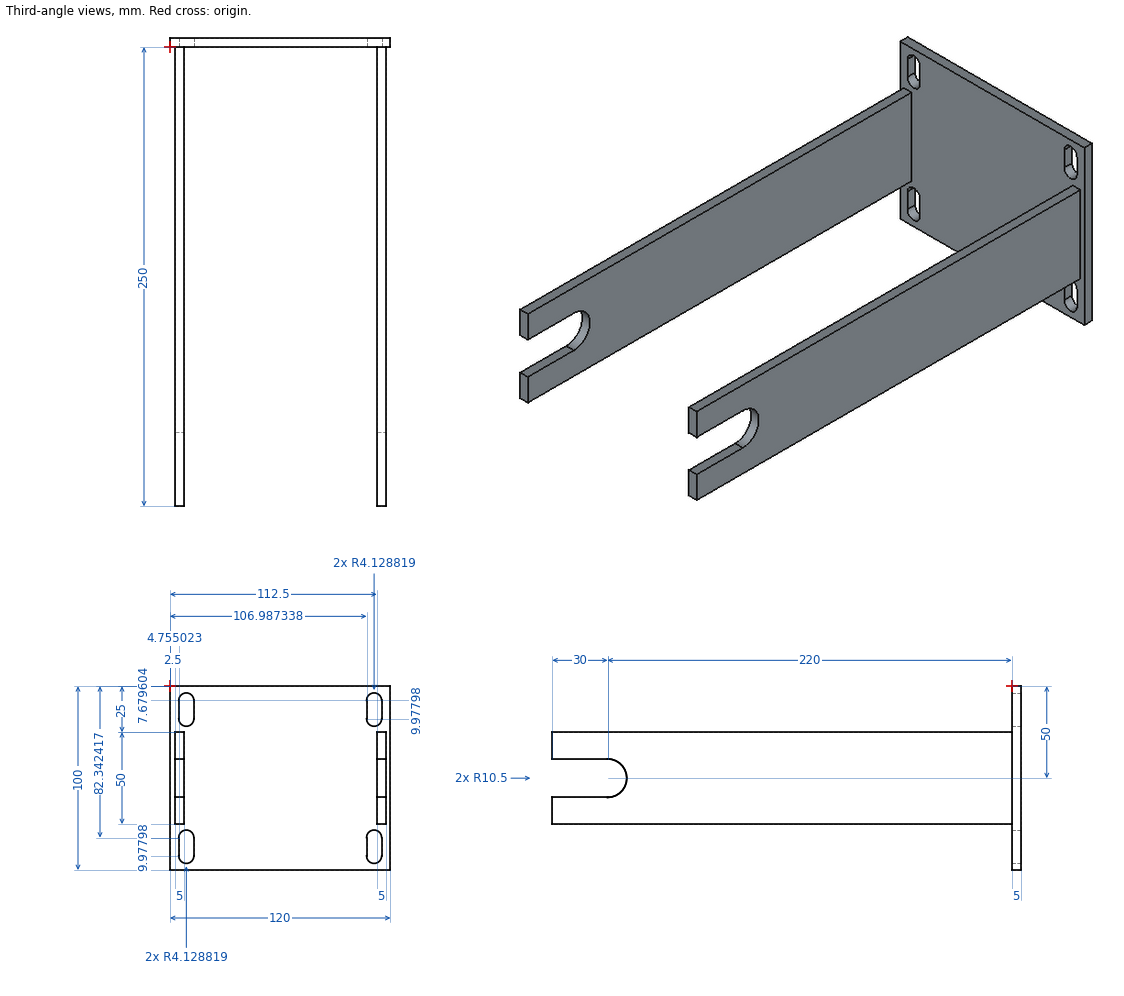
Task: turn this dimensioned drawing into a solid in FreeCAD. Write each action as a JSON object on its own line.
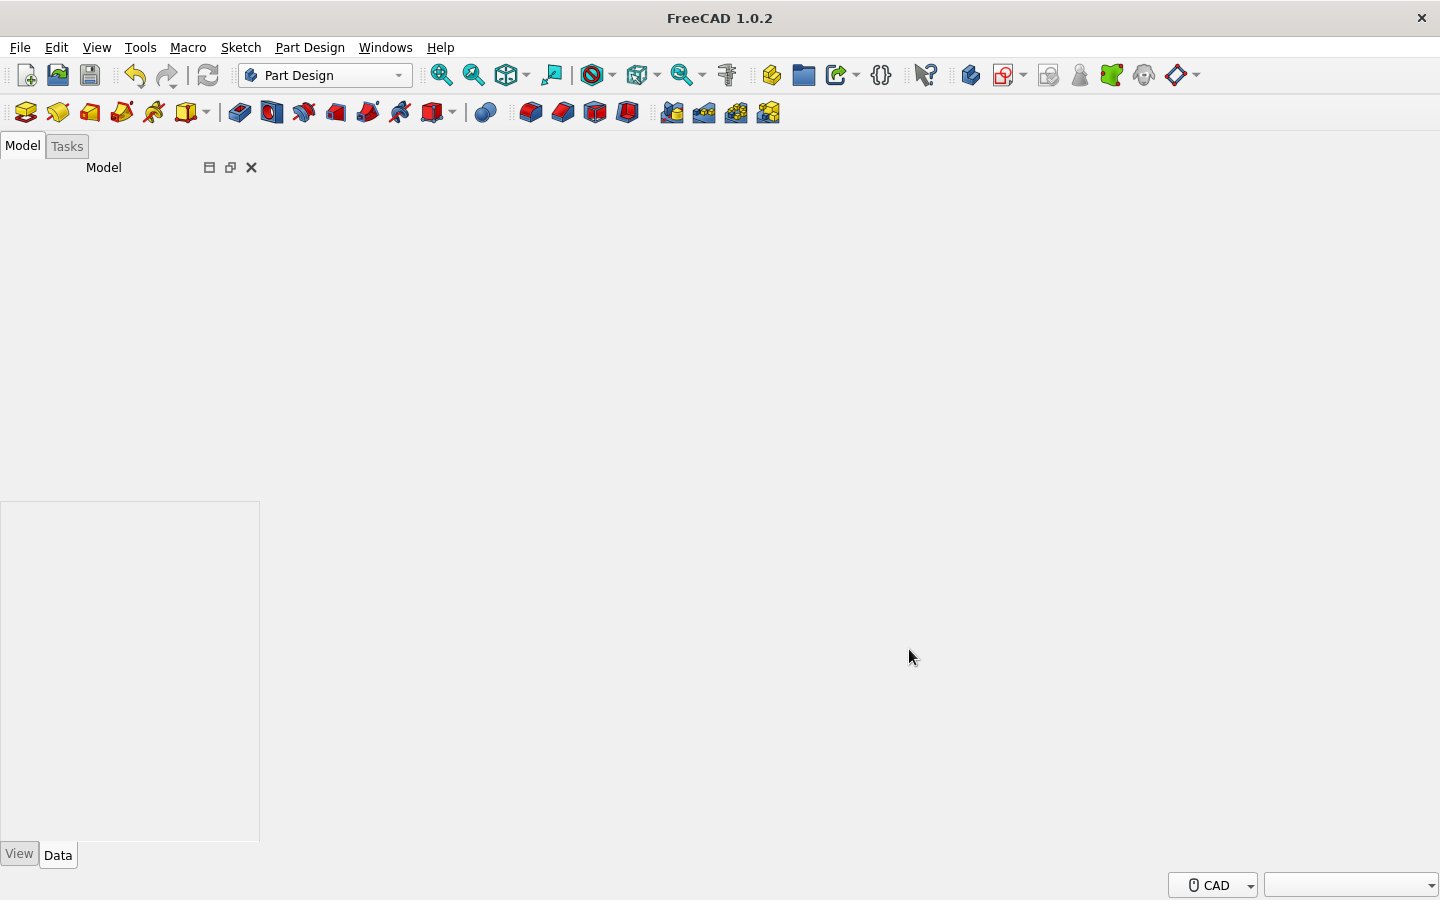
{"action": "left_click", "coordinate": [26, 76]}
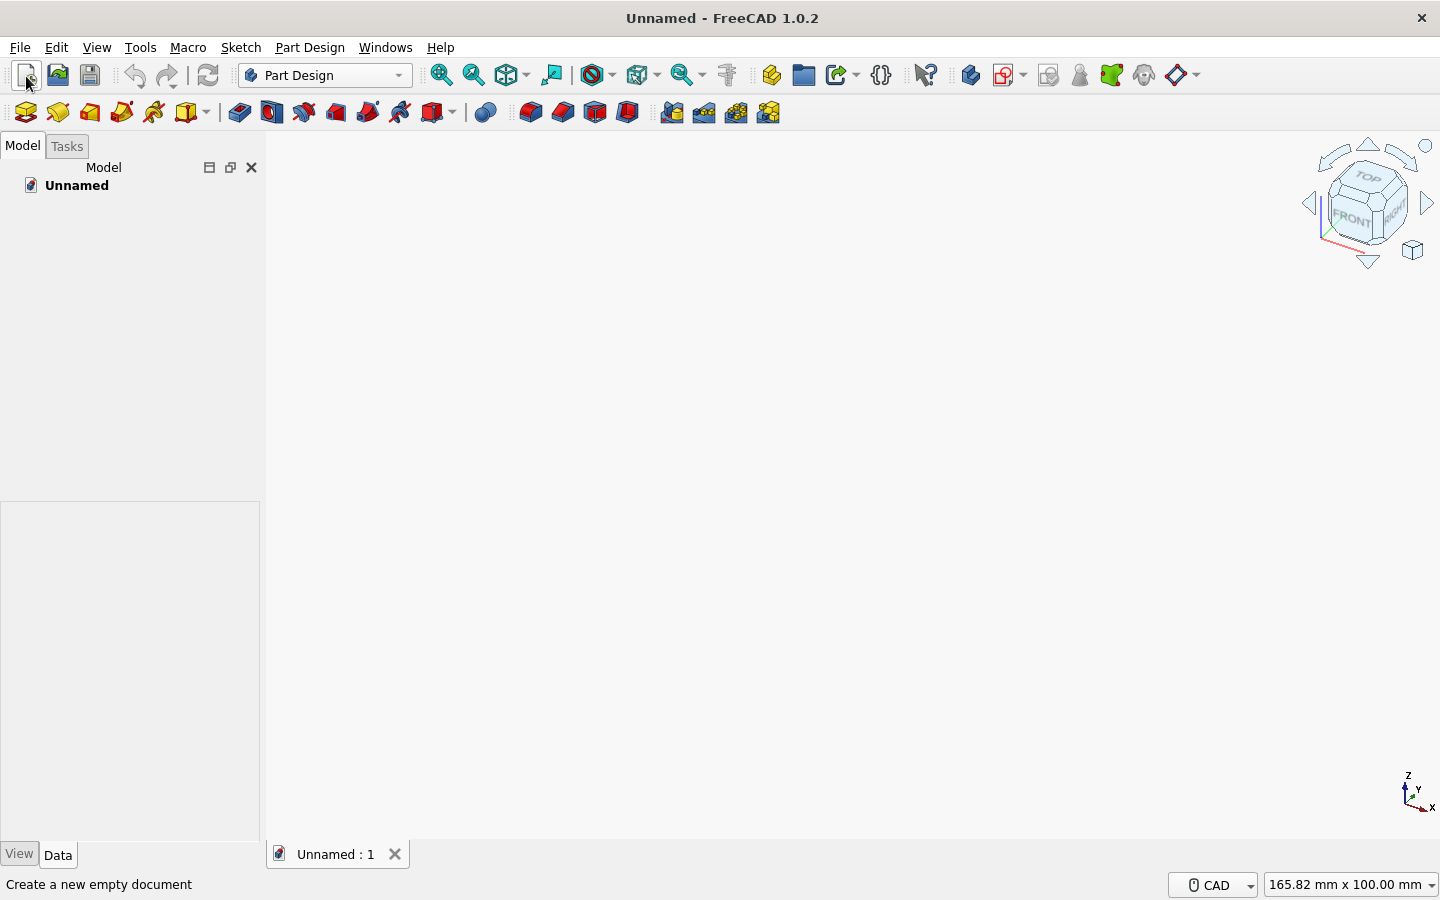
{"action": "left_click", "coordinate": [1004, 76]}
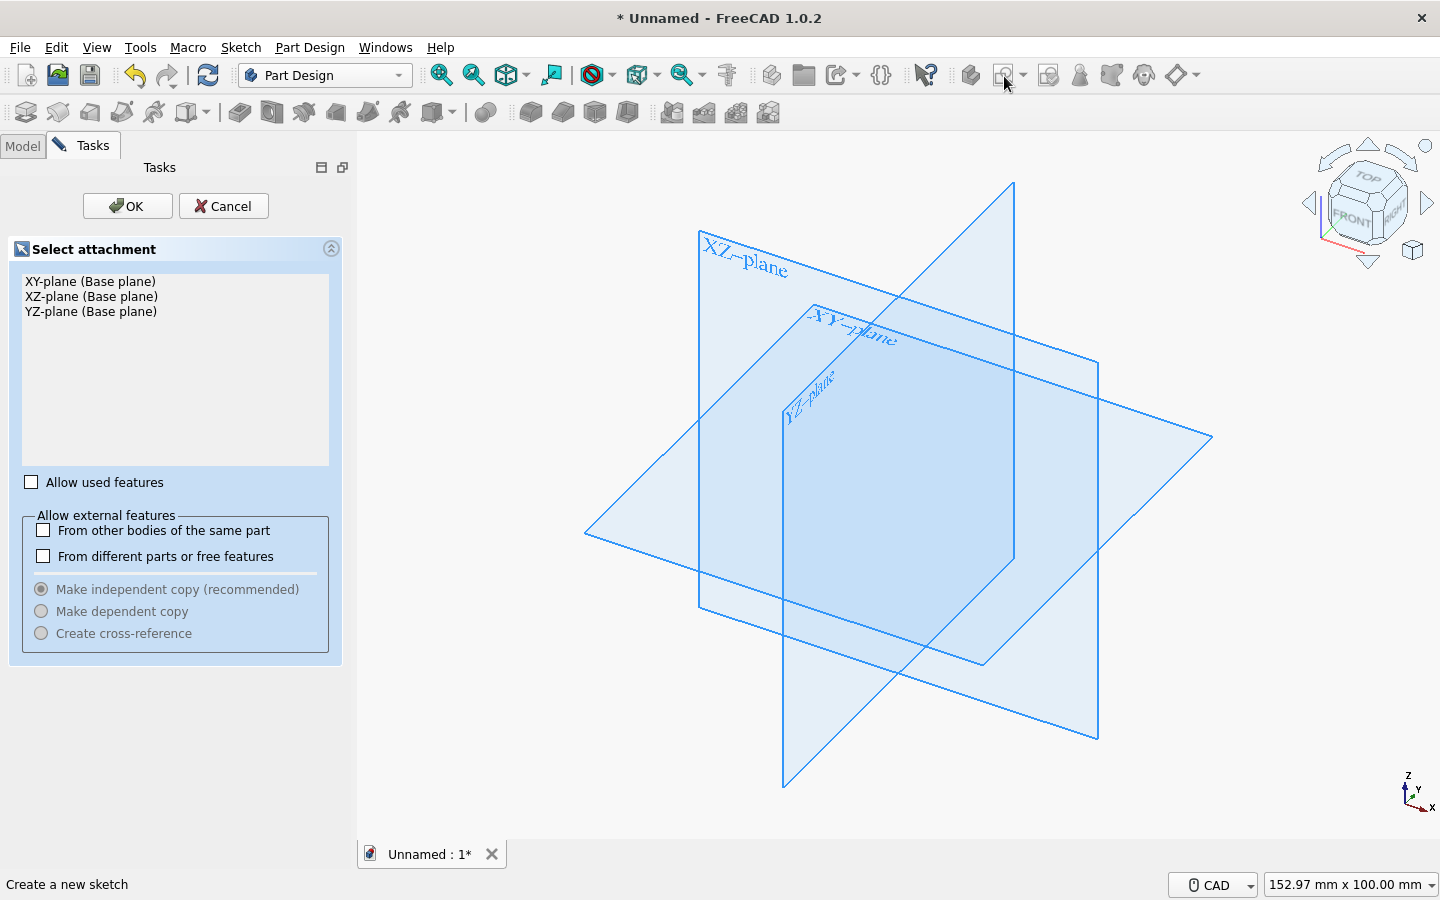
{"action": "left_click", "coordinate": [82, 296]}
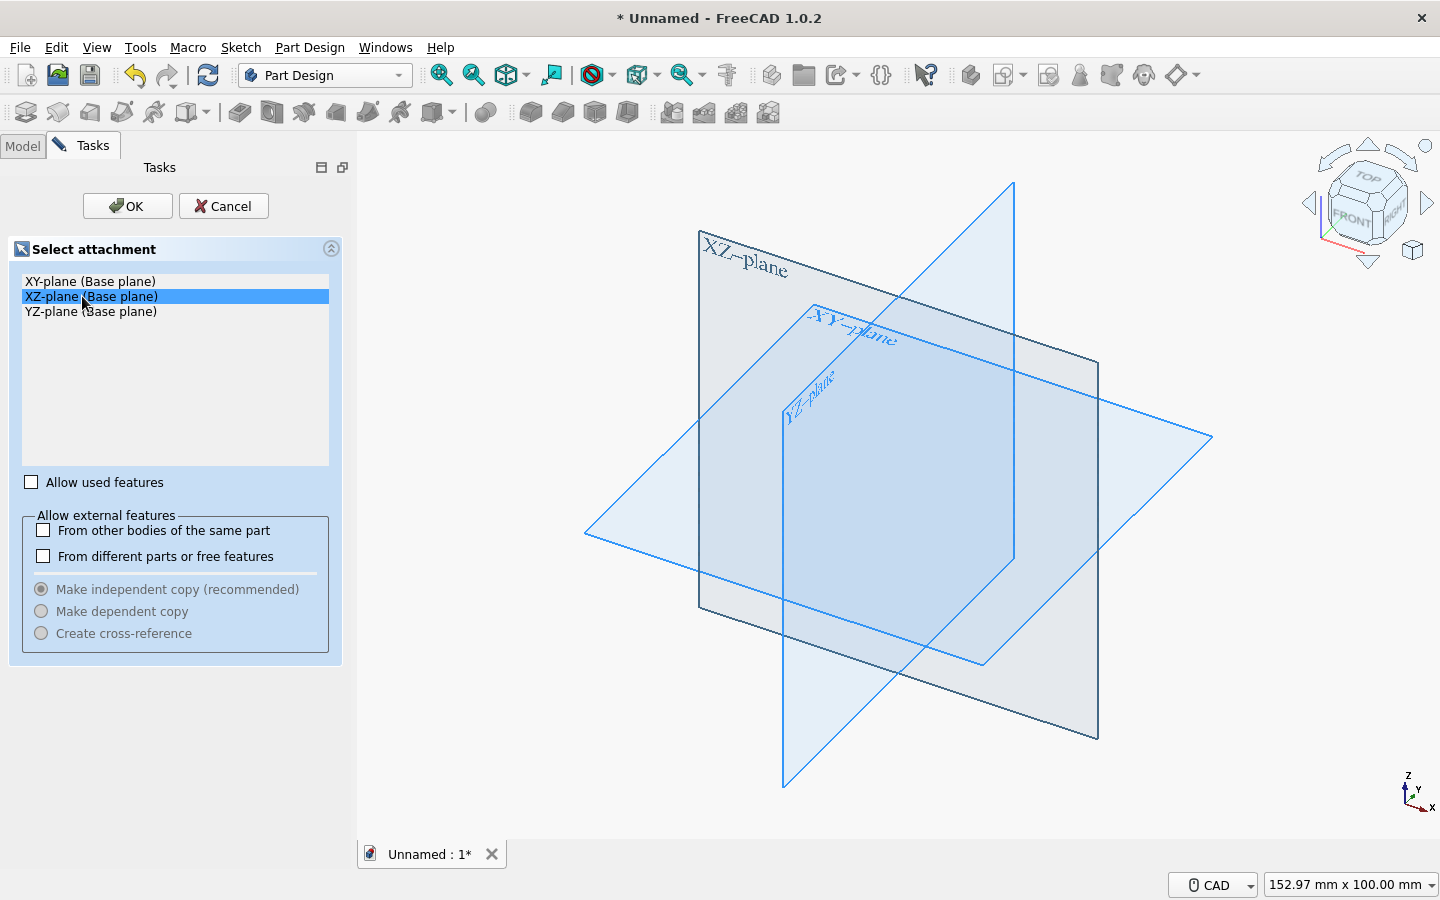
{"action": "left_click", "coordinate": [128, 206]}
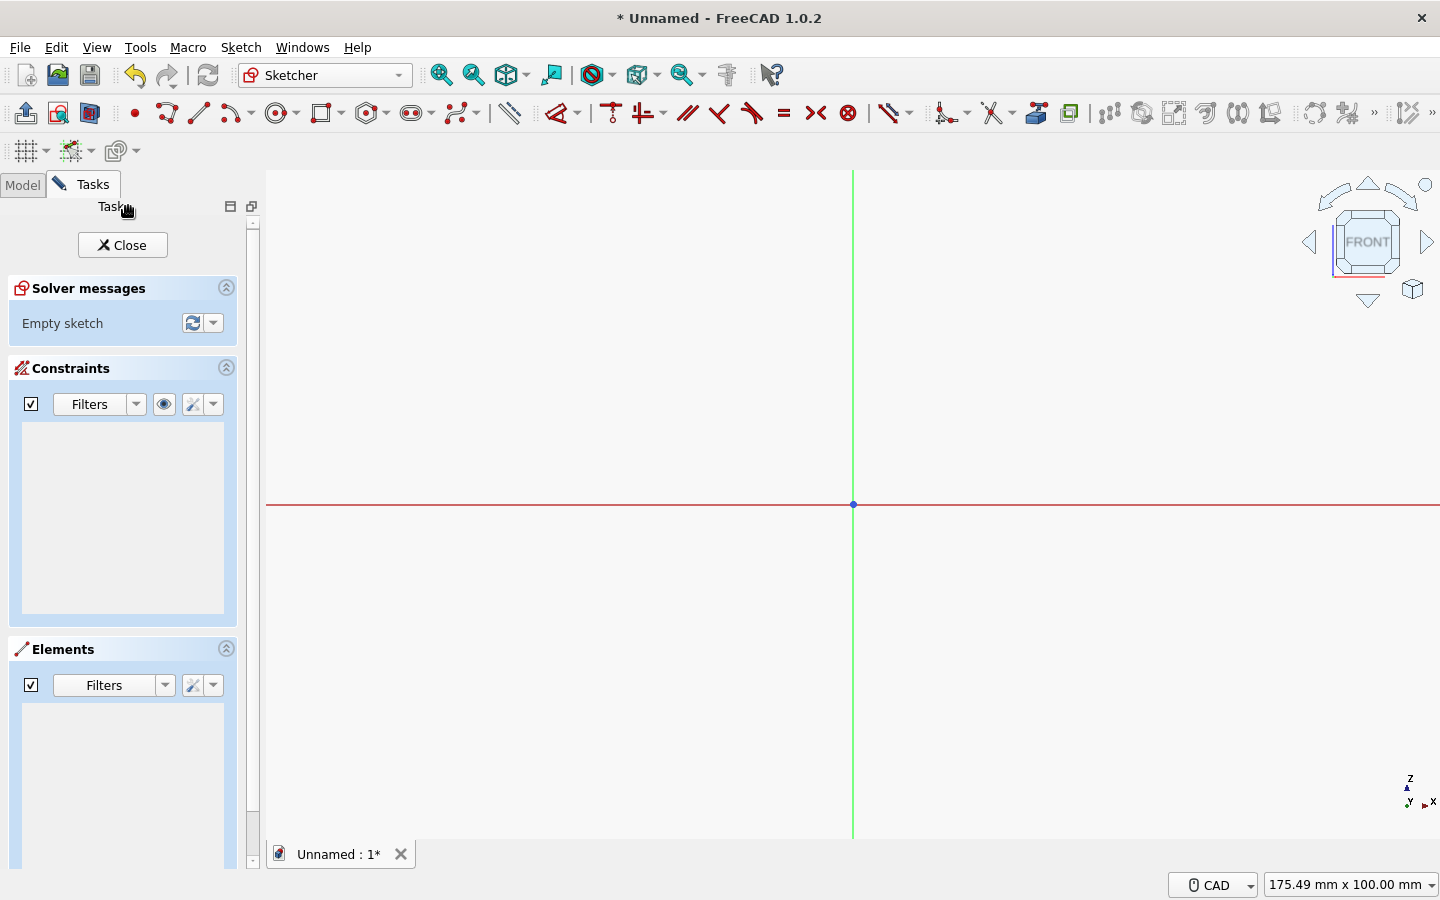
{"action": "scroll", "coordinate": [294, 198], "scroll_direction": "down", "scroll_amount": 3}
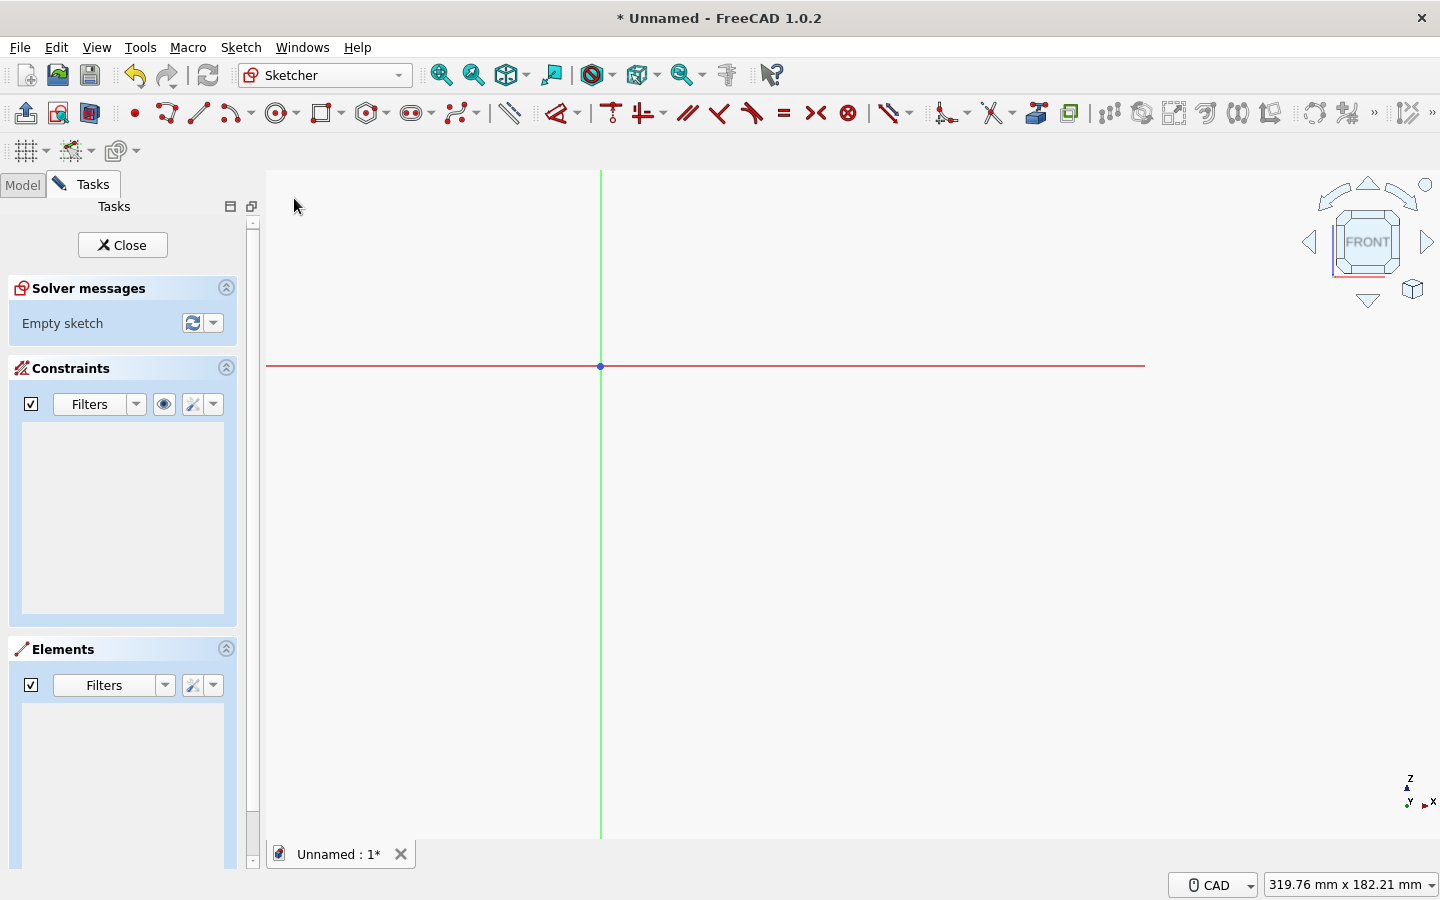
{"action": "left_click", "coordinate": [322, 114]}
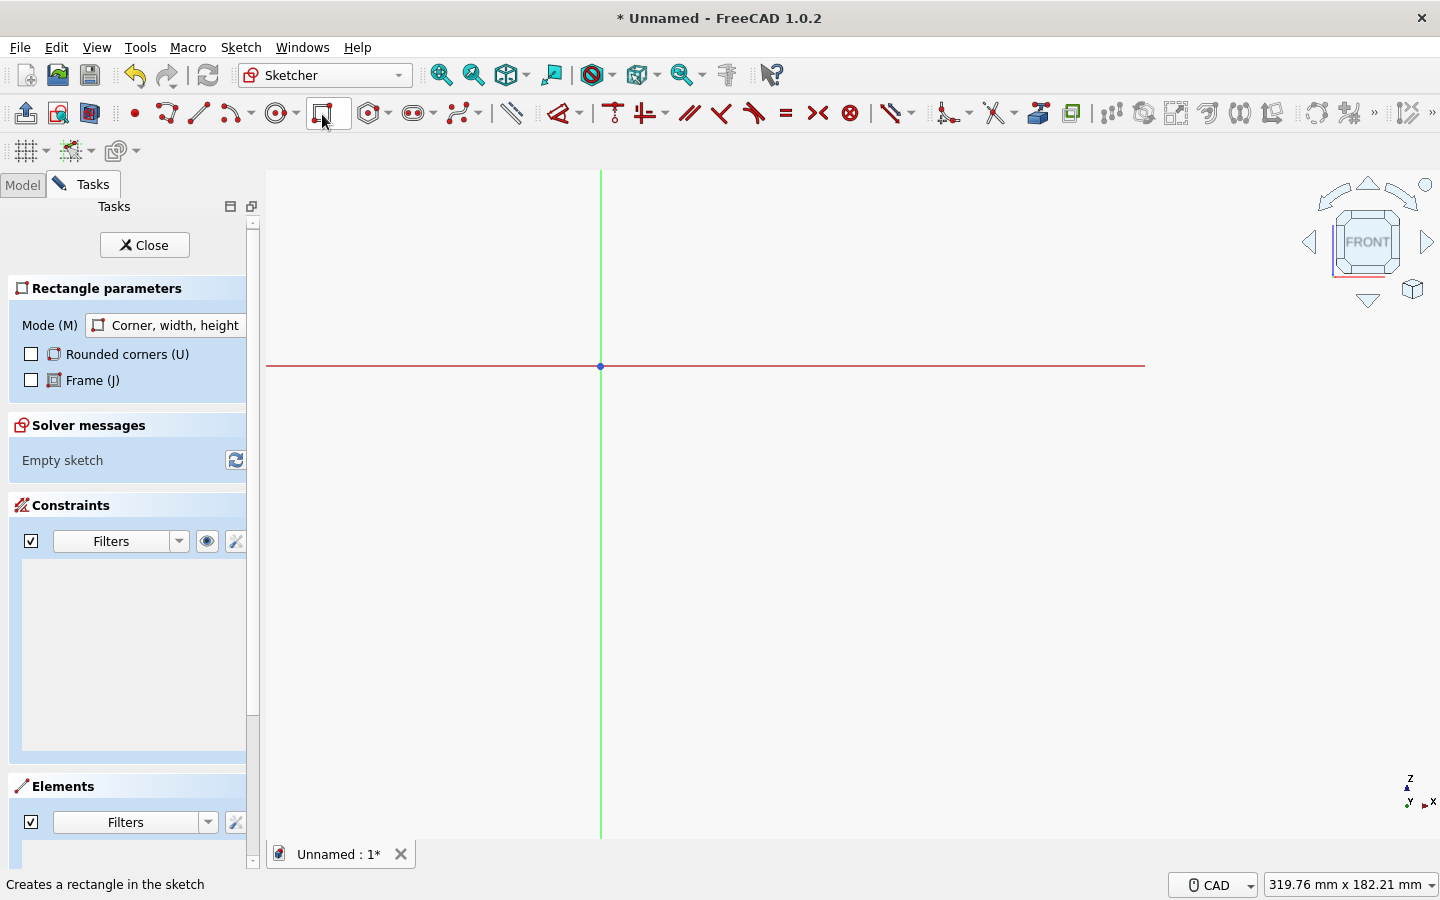
{"action": "left_click", "coordinate": [601, 366]}
{"action": "left_click", "coordinate": [1041, 733]}
{"action": "key", "text": "Escape"}